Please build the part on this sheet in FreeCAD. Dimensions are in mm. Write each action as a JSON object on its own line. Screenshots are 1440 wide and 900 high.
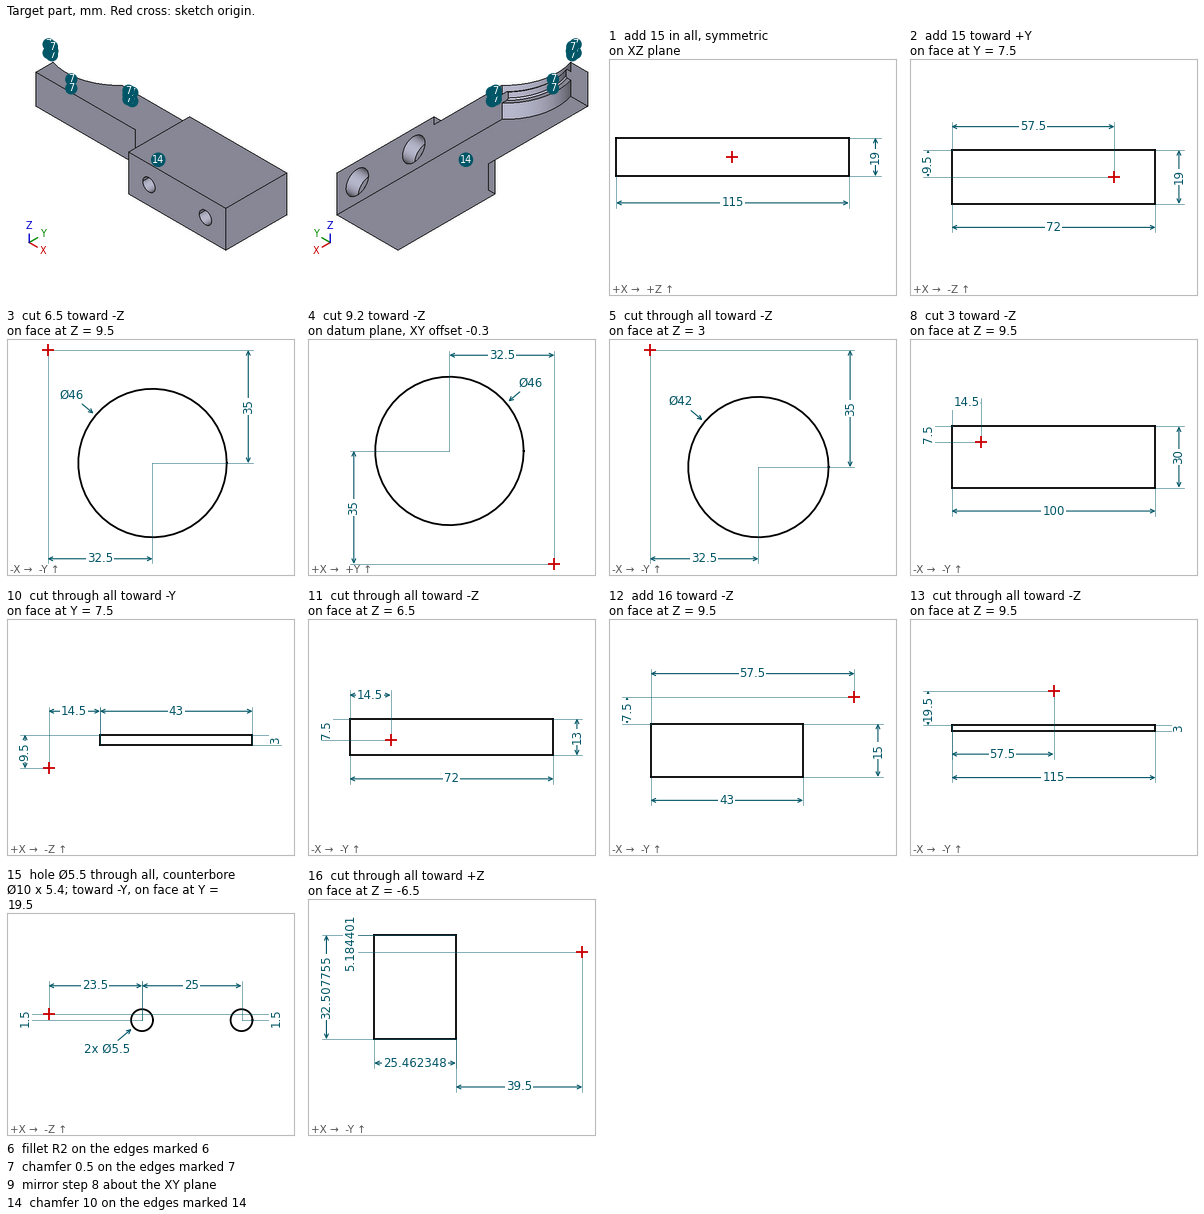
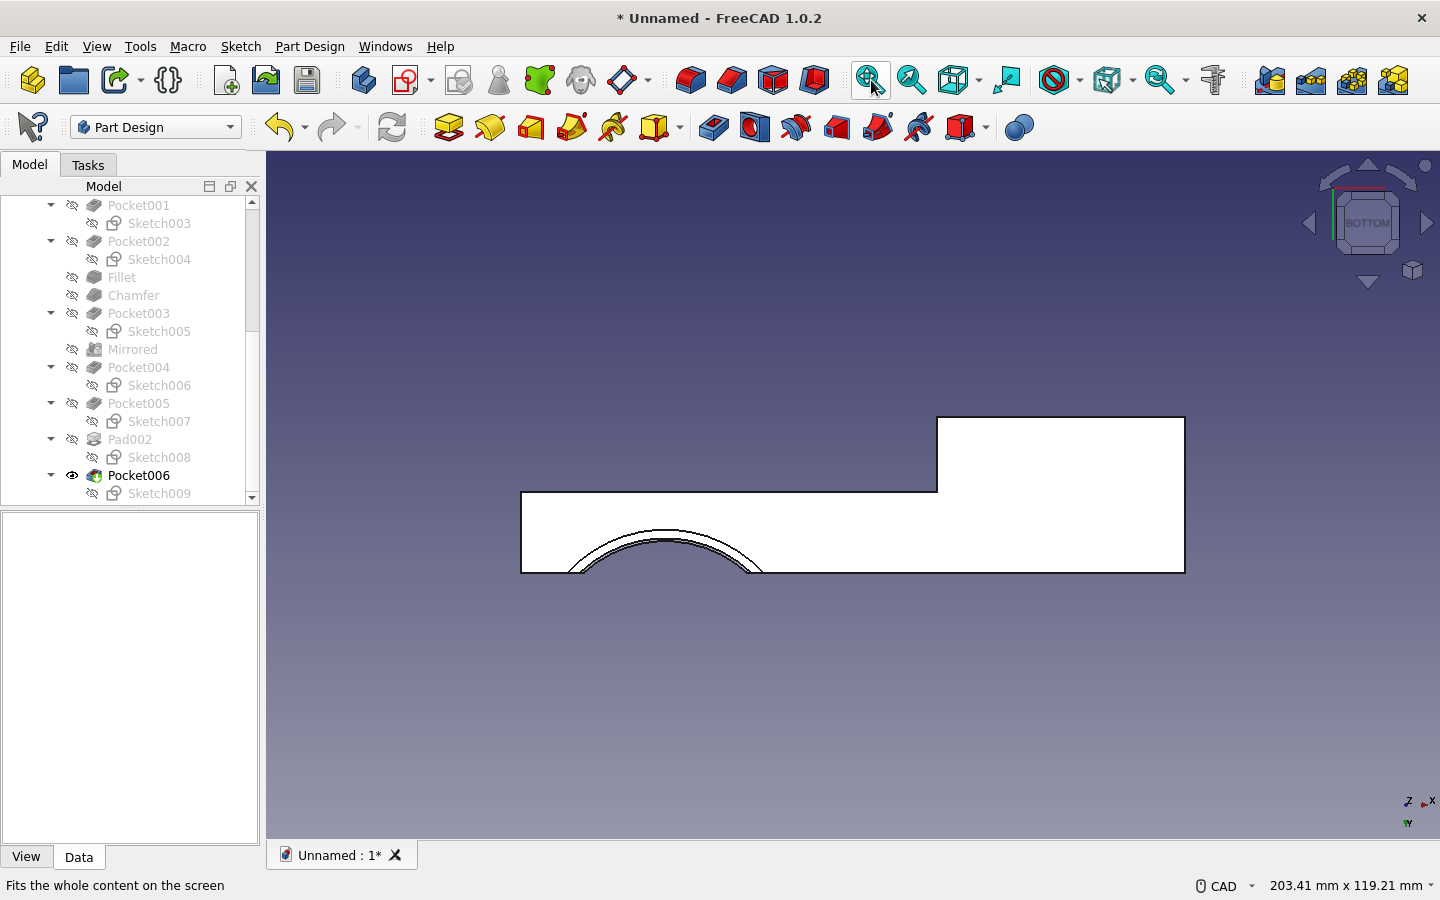
{"action": "key", "text": "4"}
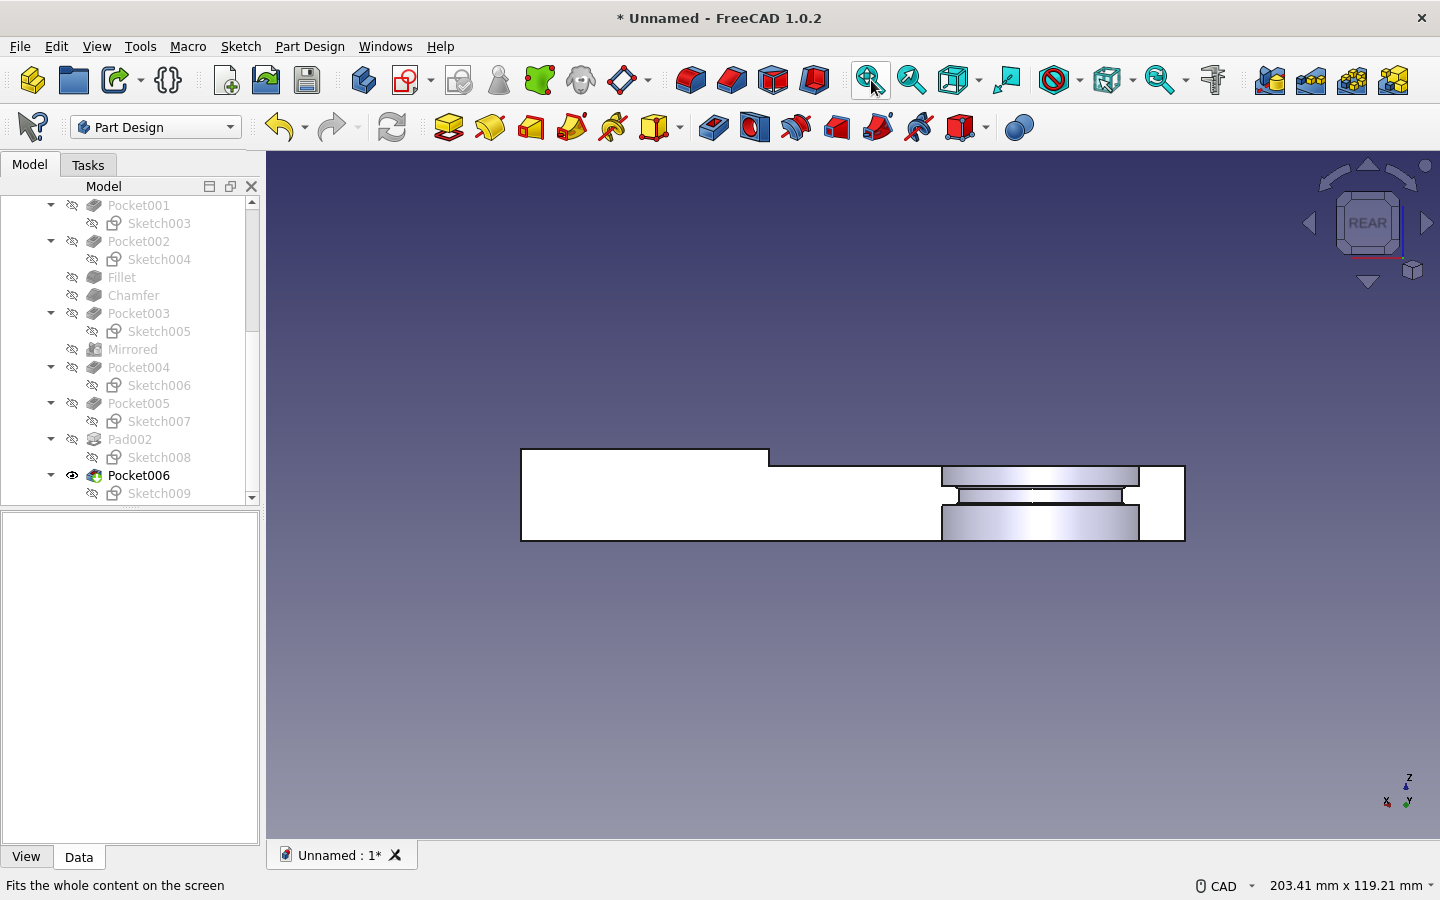
{"action": "key", "text": "6"}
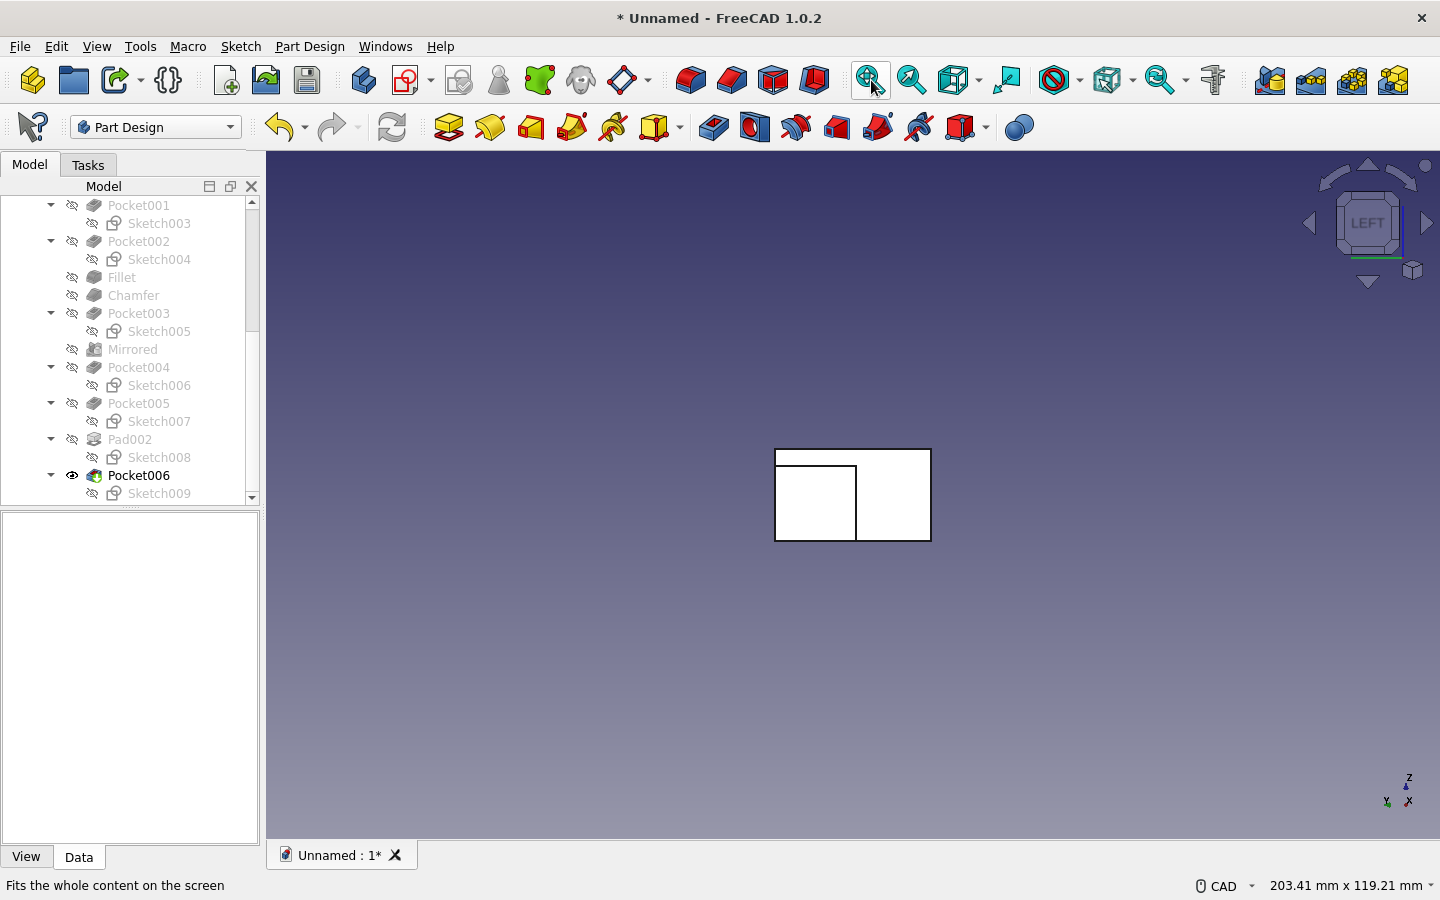
{"action": "left_click", "coordinate": [871, 80]}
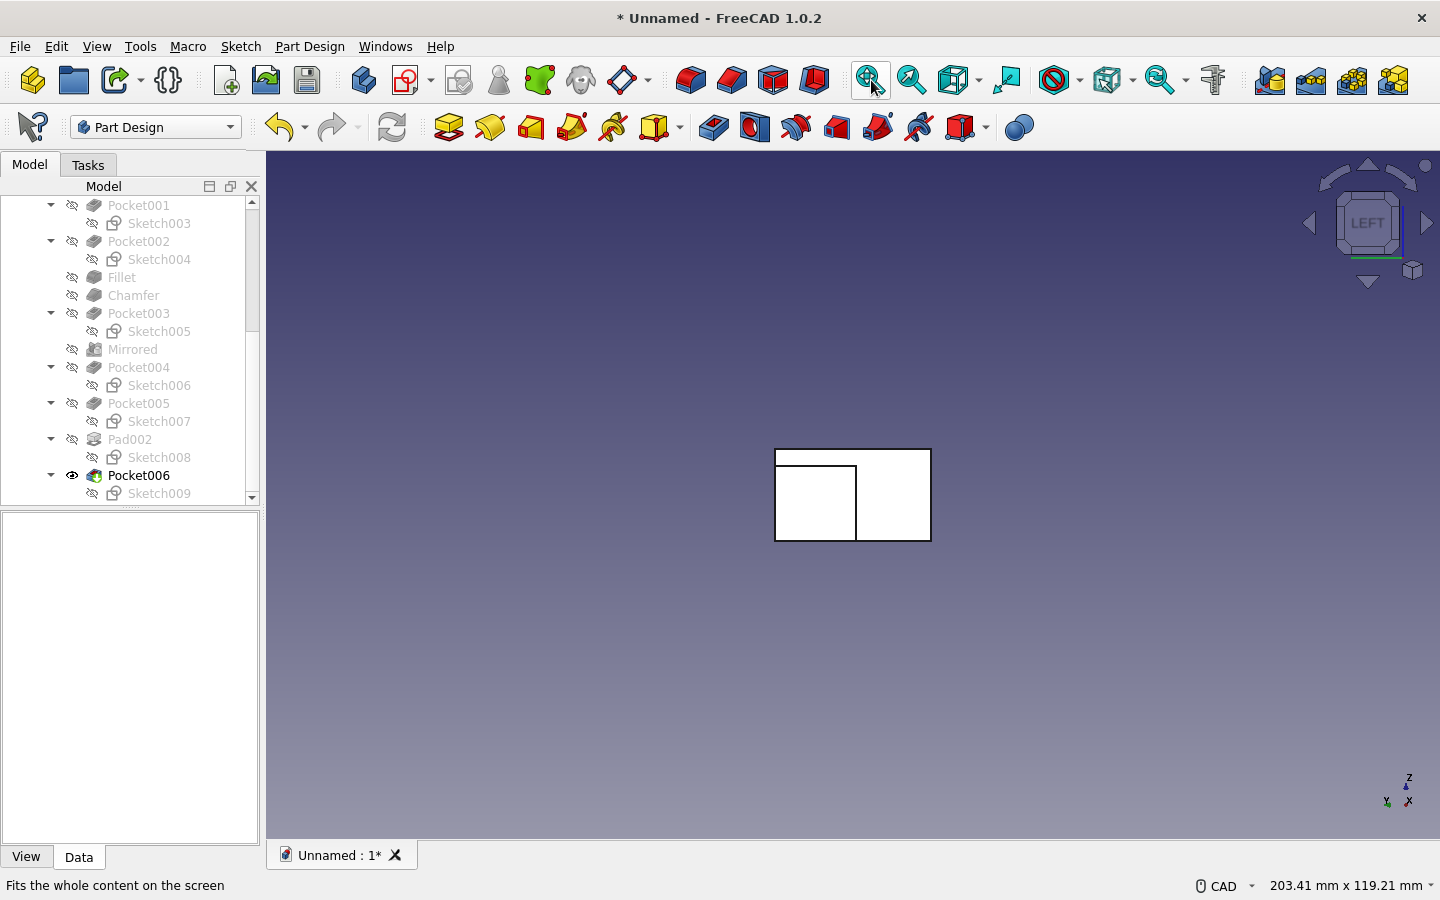
{"action": "key", "text": "v 3"}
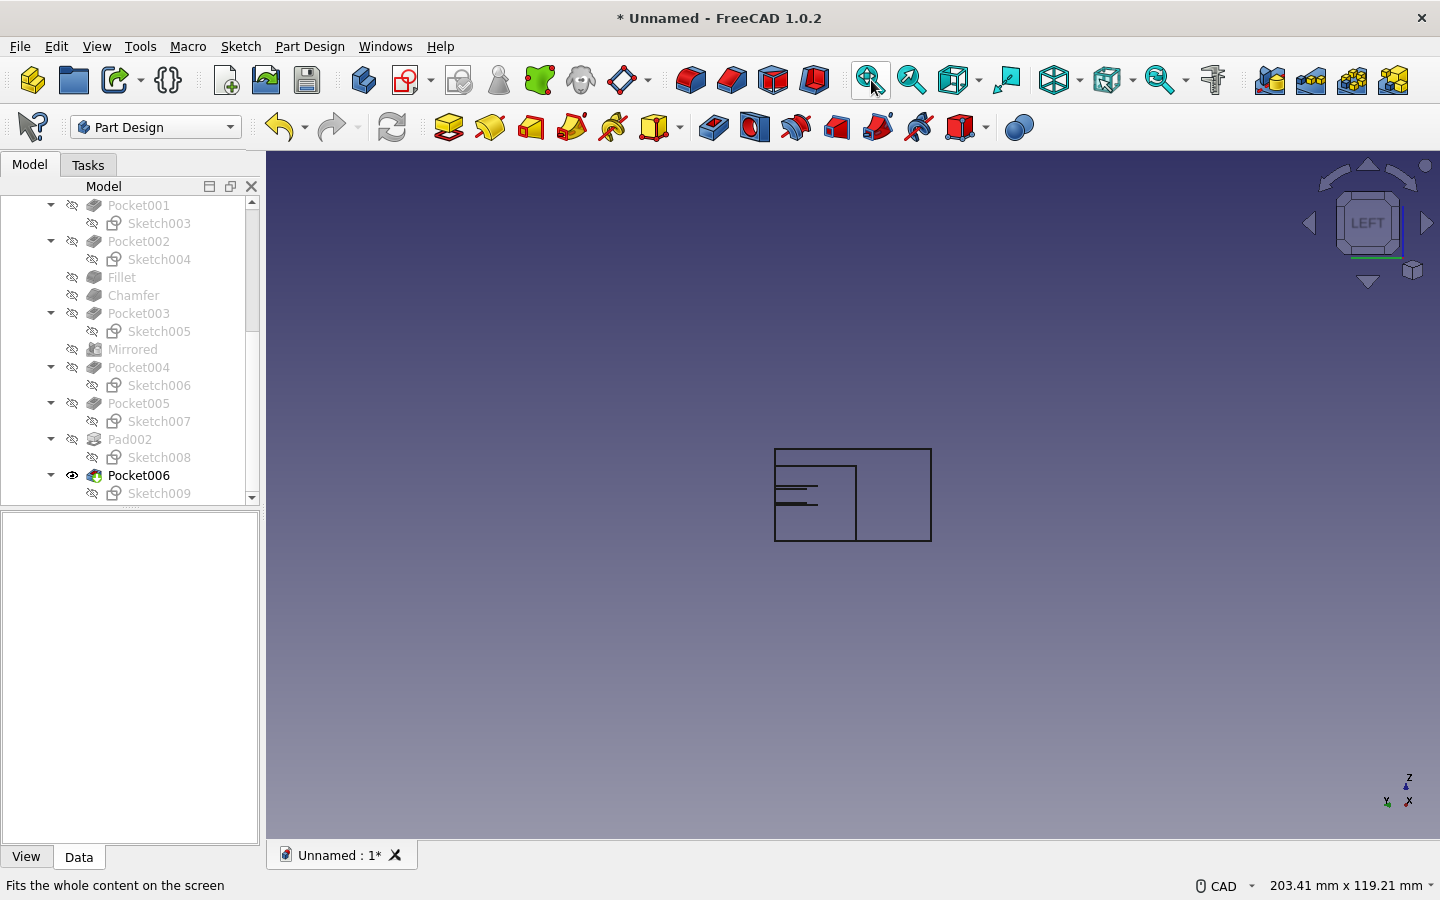
{"action": "key", "text": "0"}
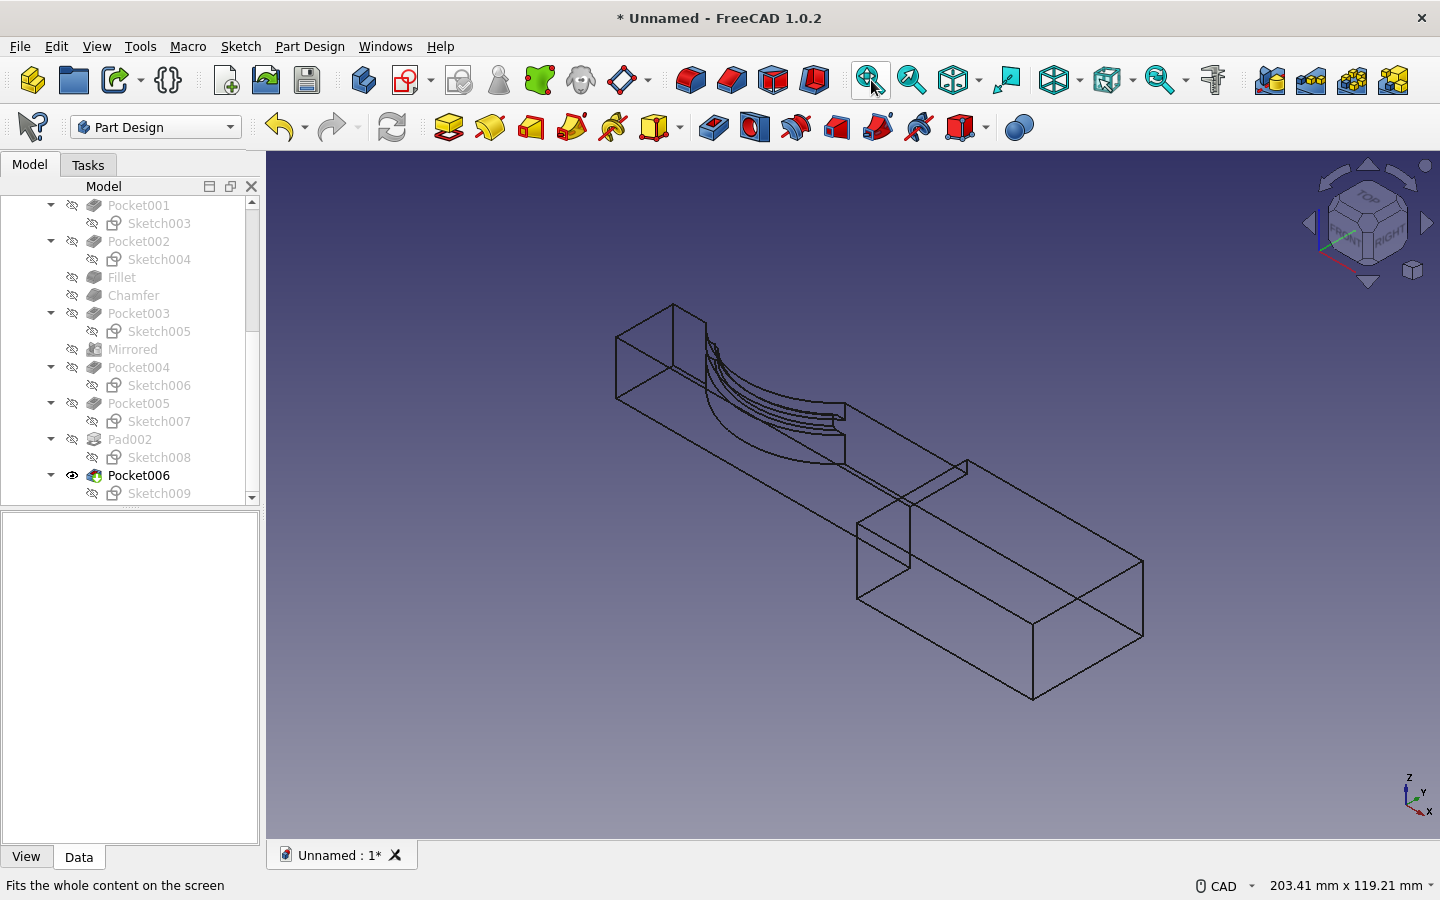
{"action": "left_click", "coordinate": [910, 536]}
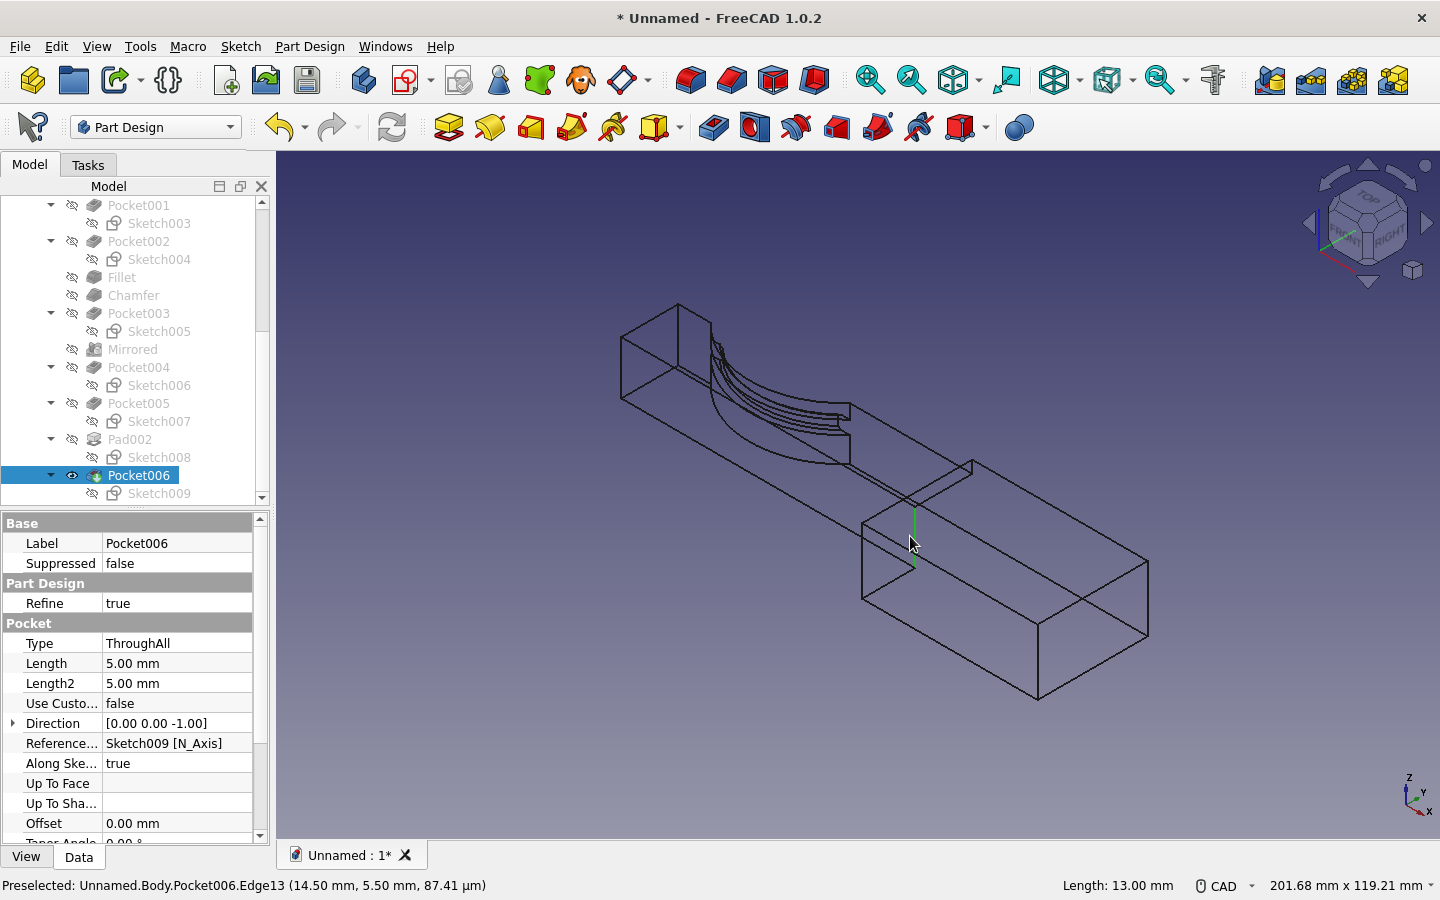
{"action": "key", "text": "v 1"}